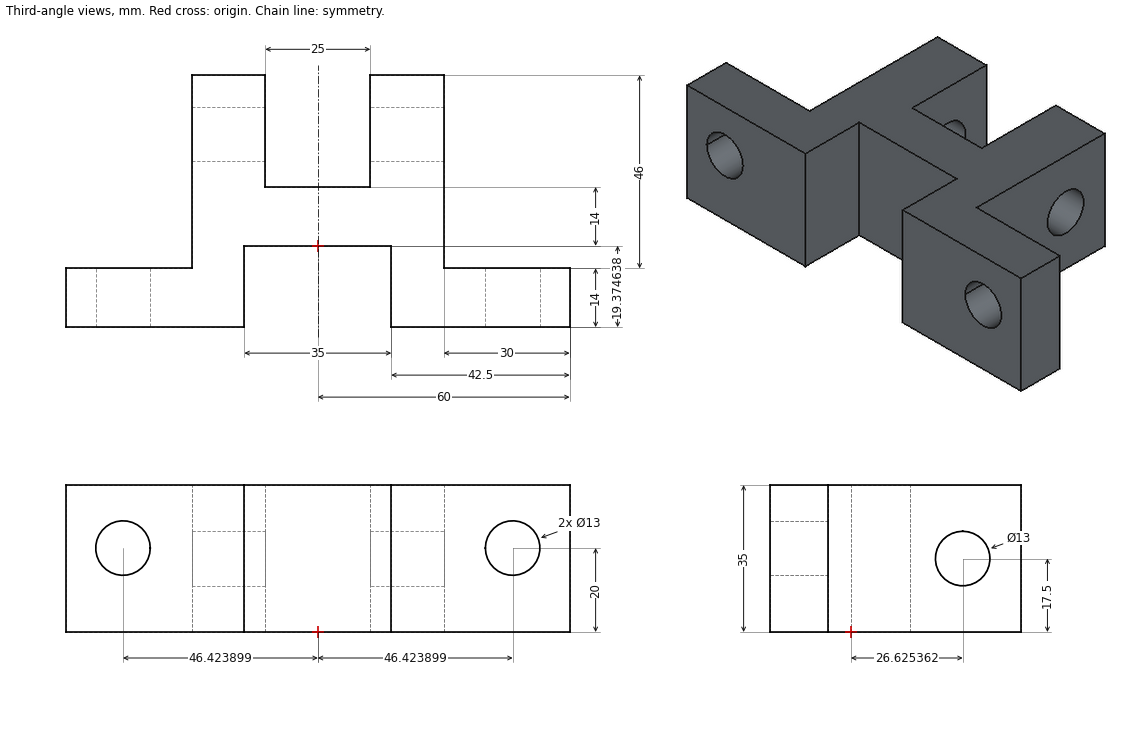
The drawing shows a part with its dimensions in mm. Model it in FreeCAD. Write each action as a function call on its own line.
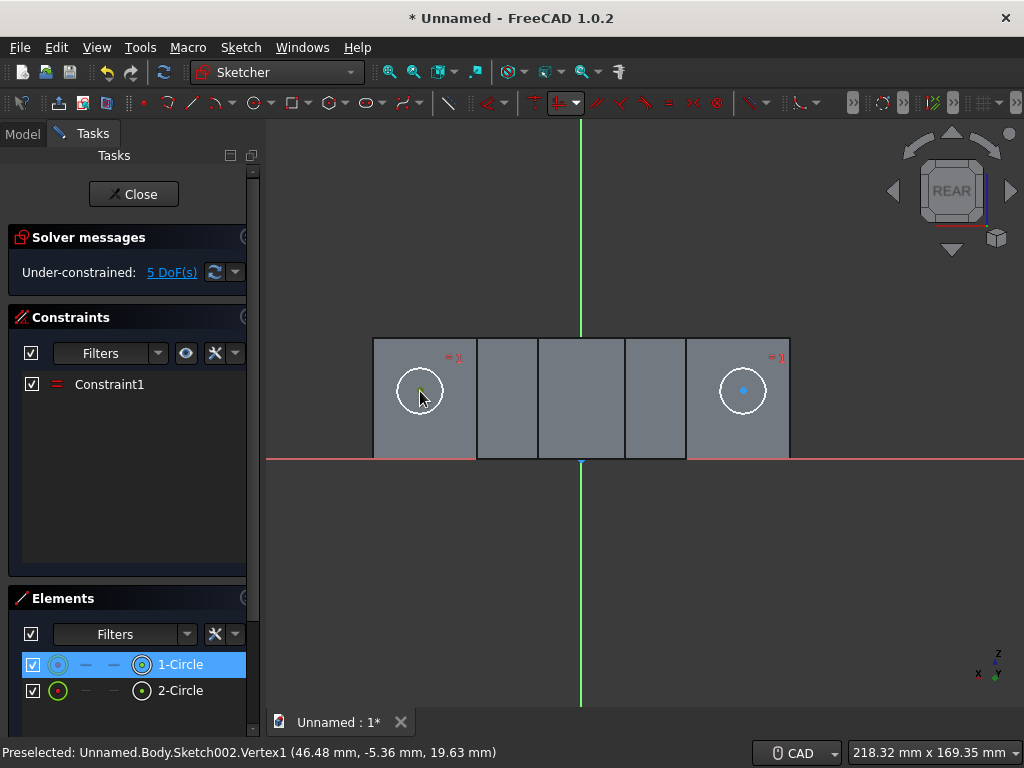
click(743, 391)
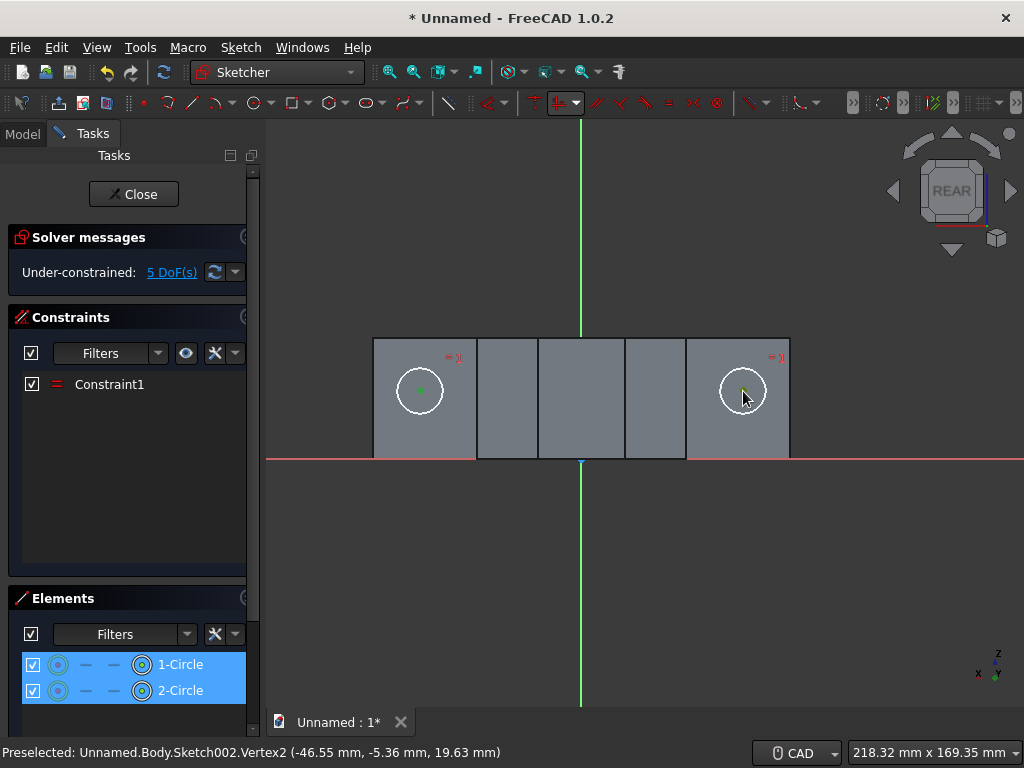
click(578, 104)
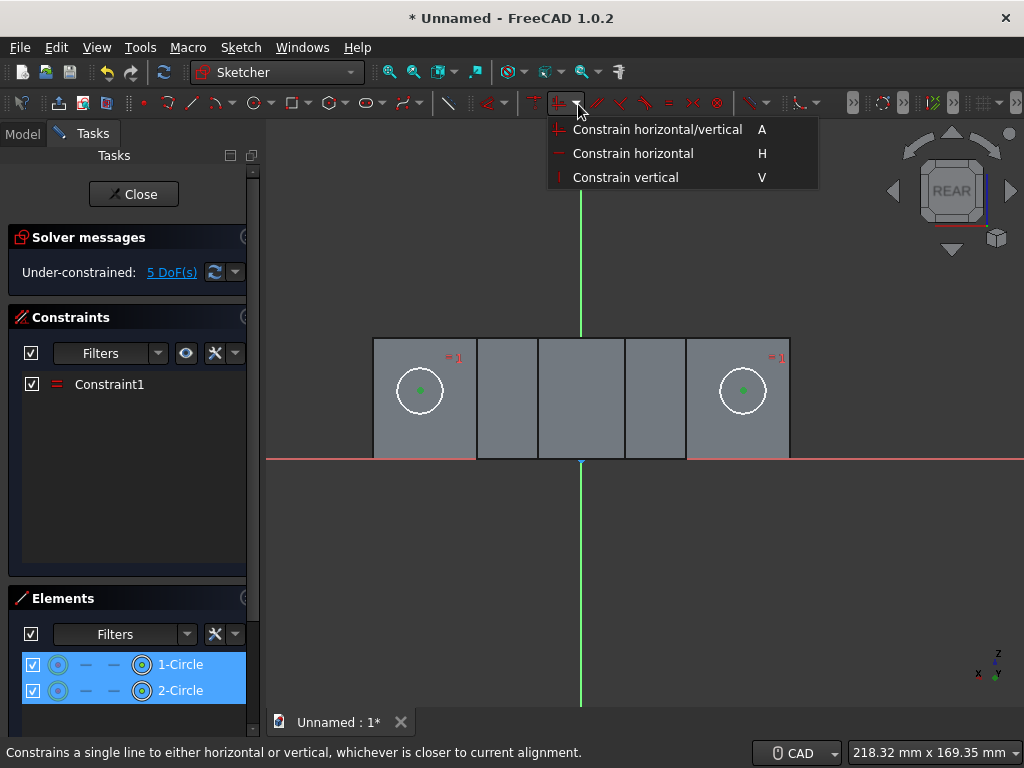
click(683, 153)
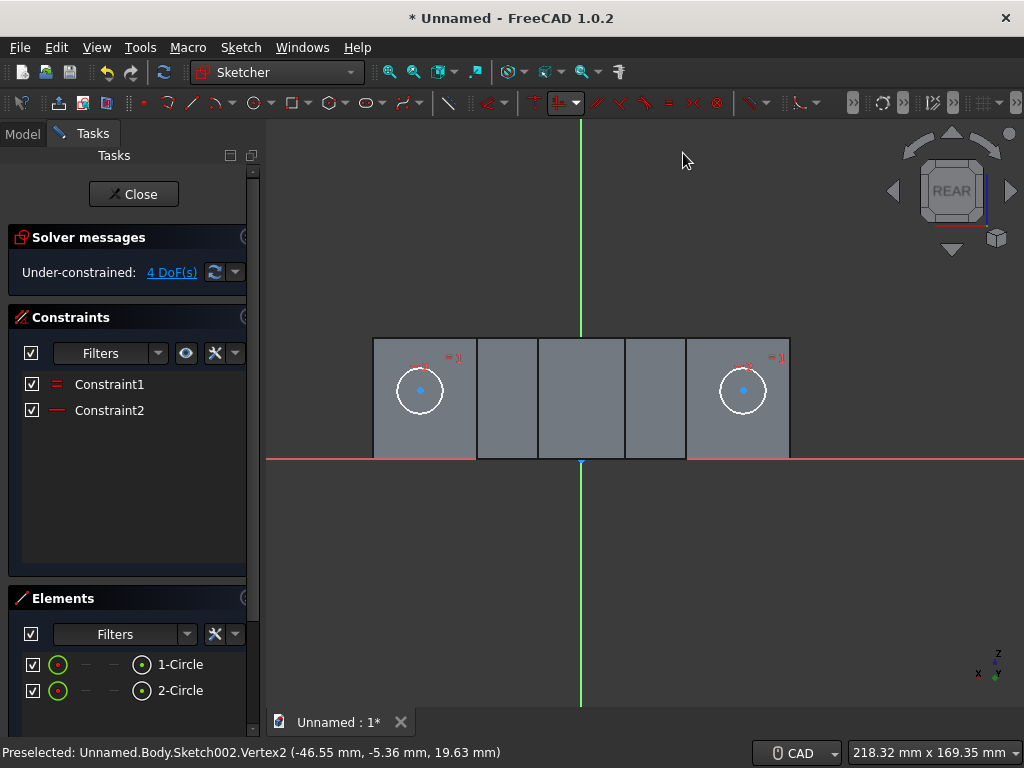
click(488, 104)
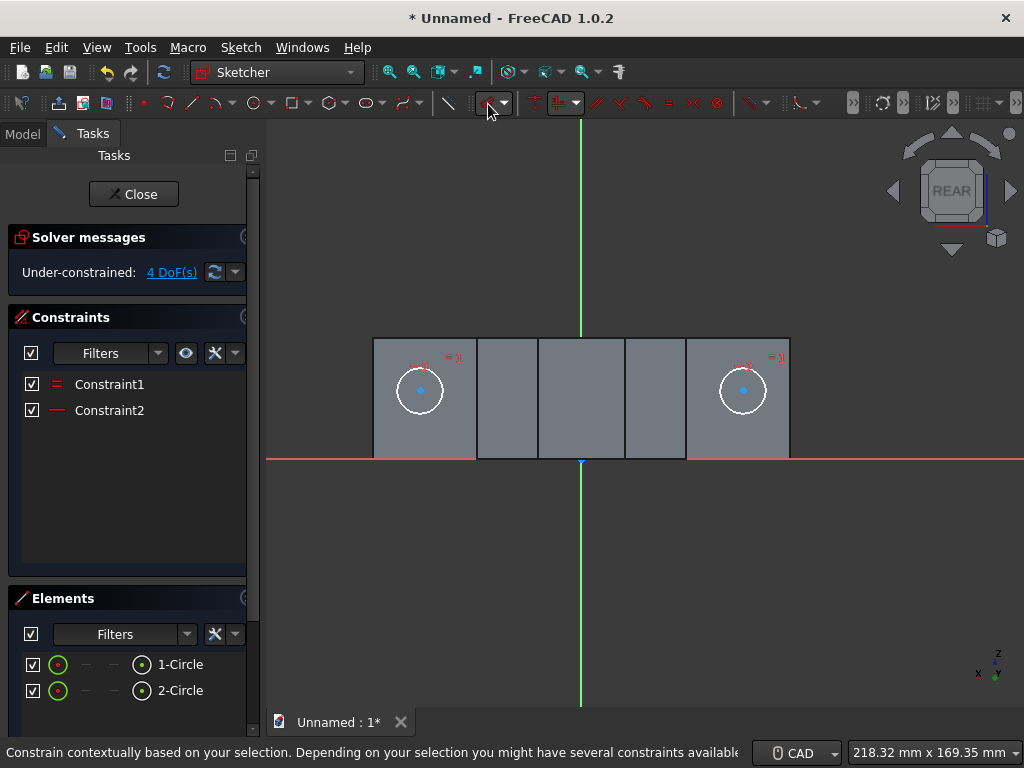
click(436, 375)
click(459, 352)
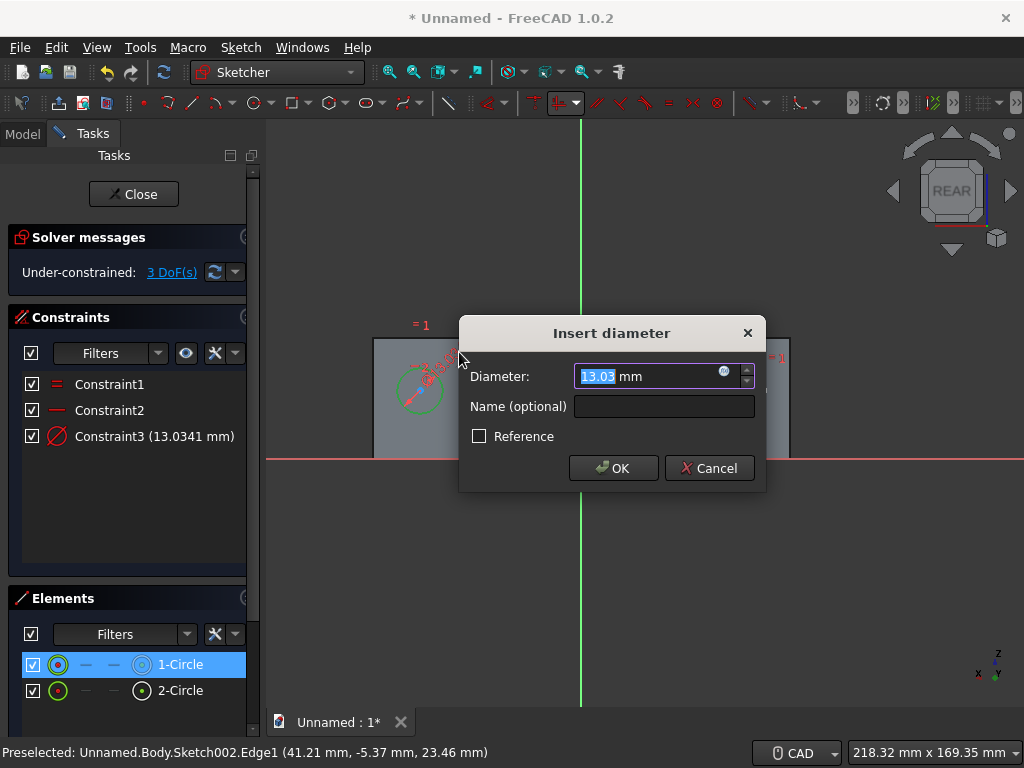
text(13)
key(Return)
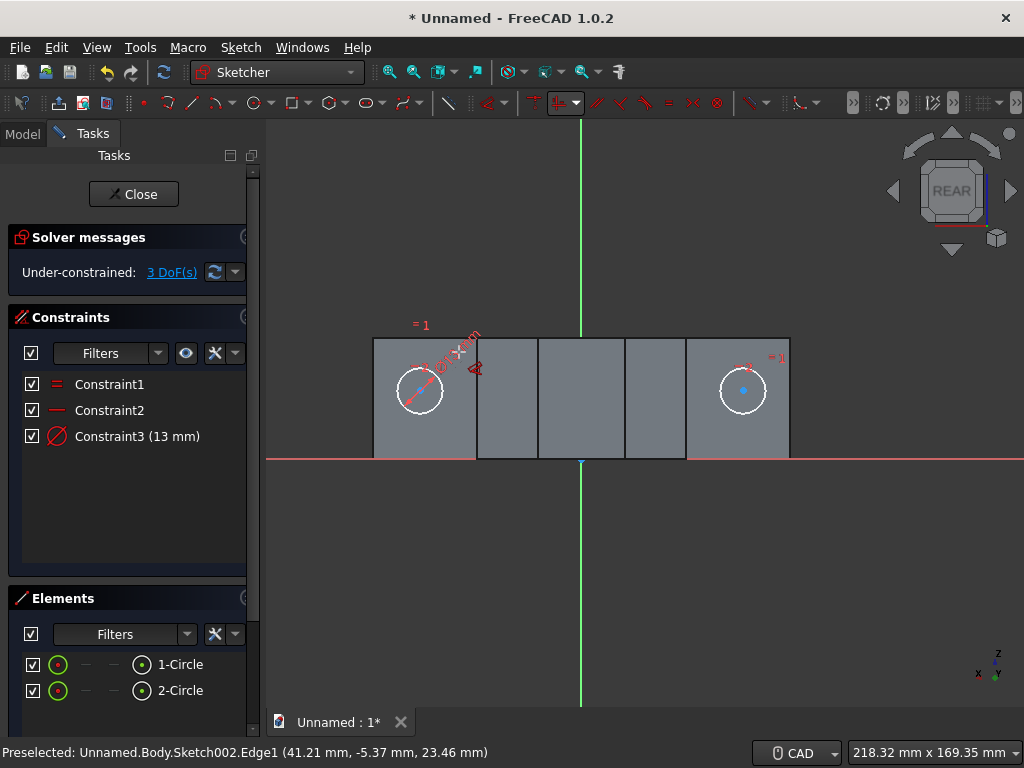
click(420, 391)
click(386, 425)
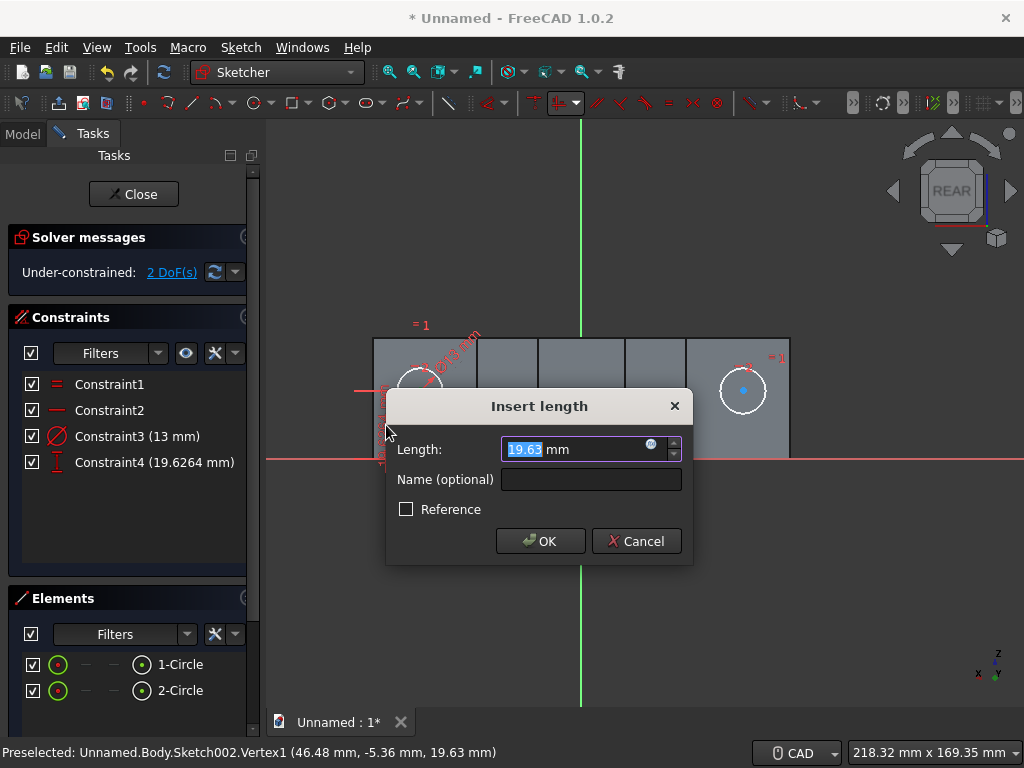
text(20)
key(Return)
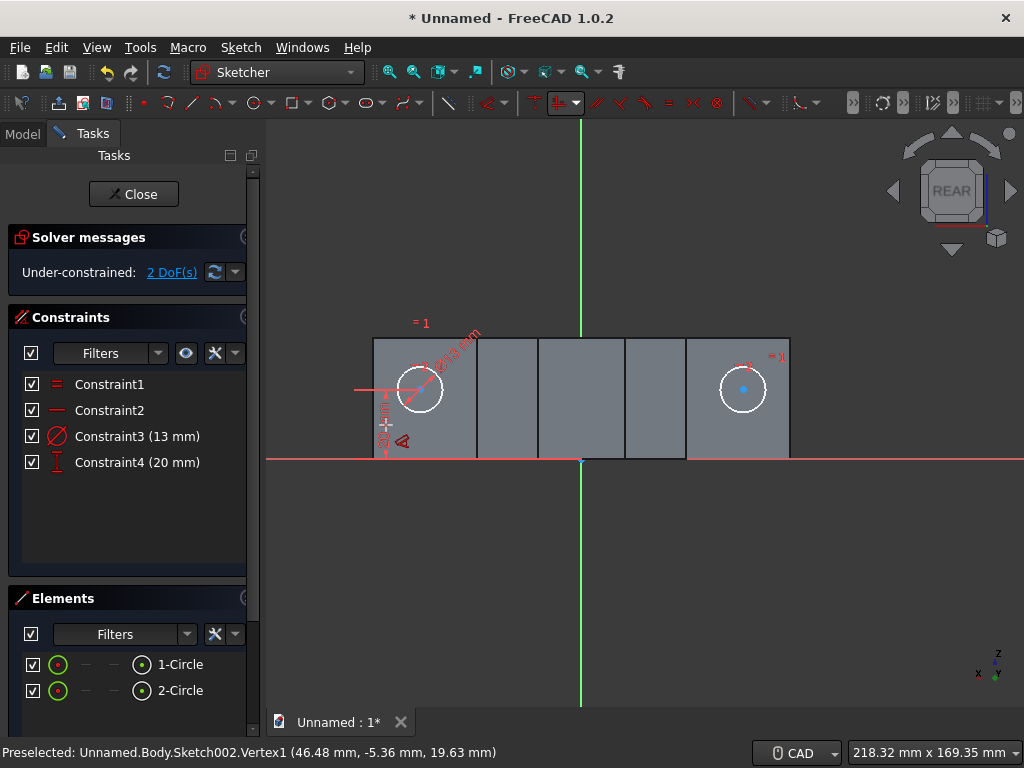
click(420, 390)
click(501, 493)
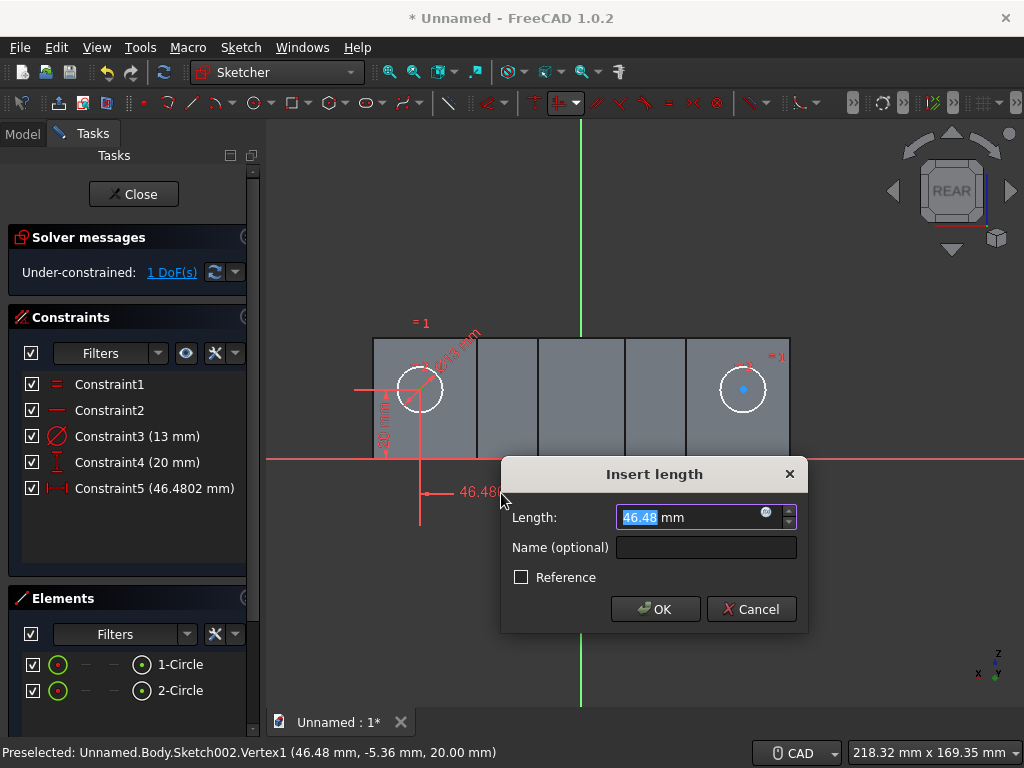
text(46.423899)
key(Return)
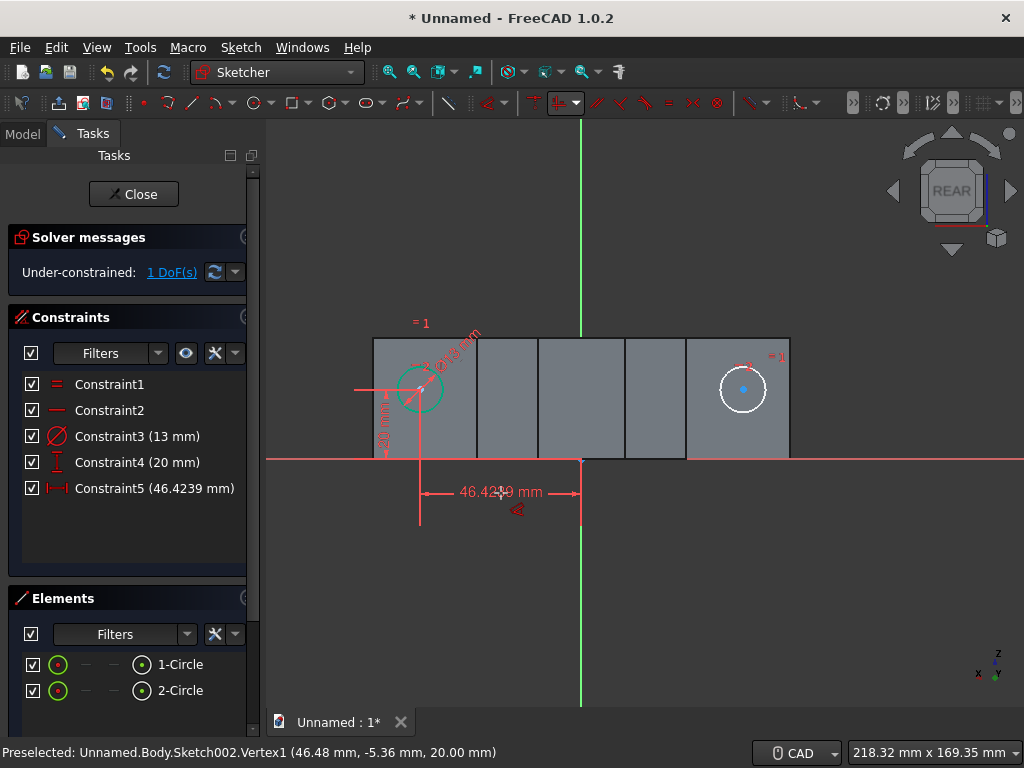
click(743, 390)
click(662, 493)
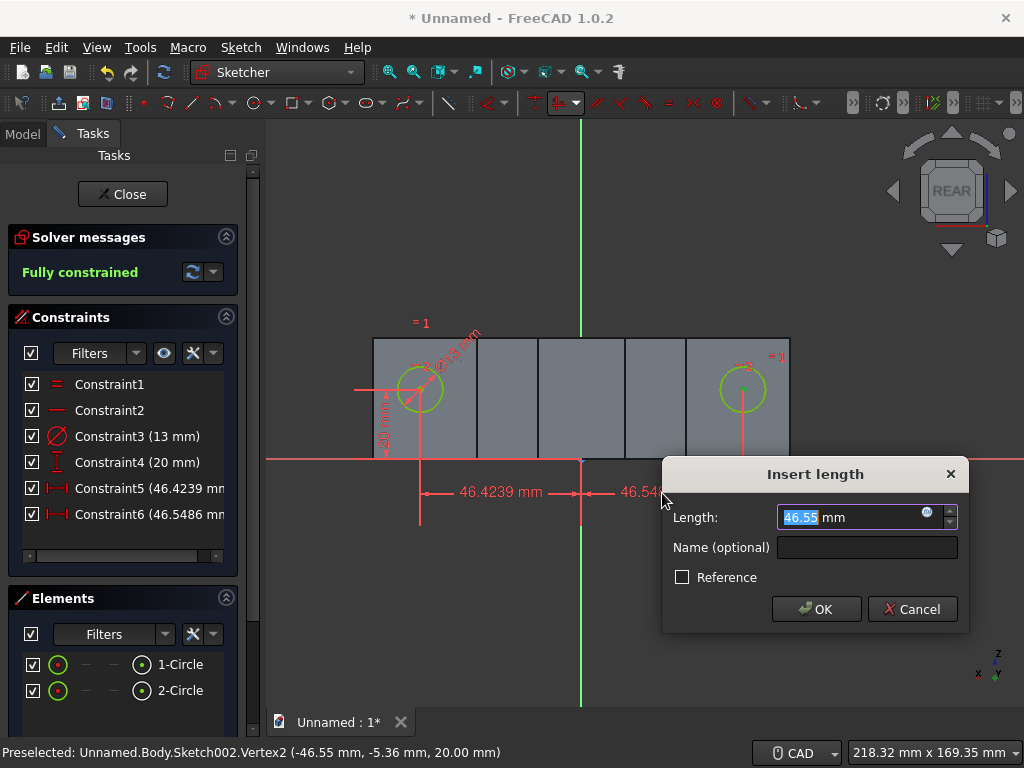
text(46.423899)
key(Return)
key(Escape)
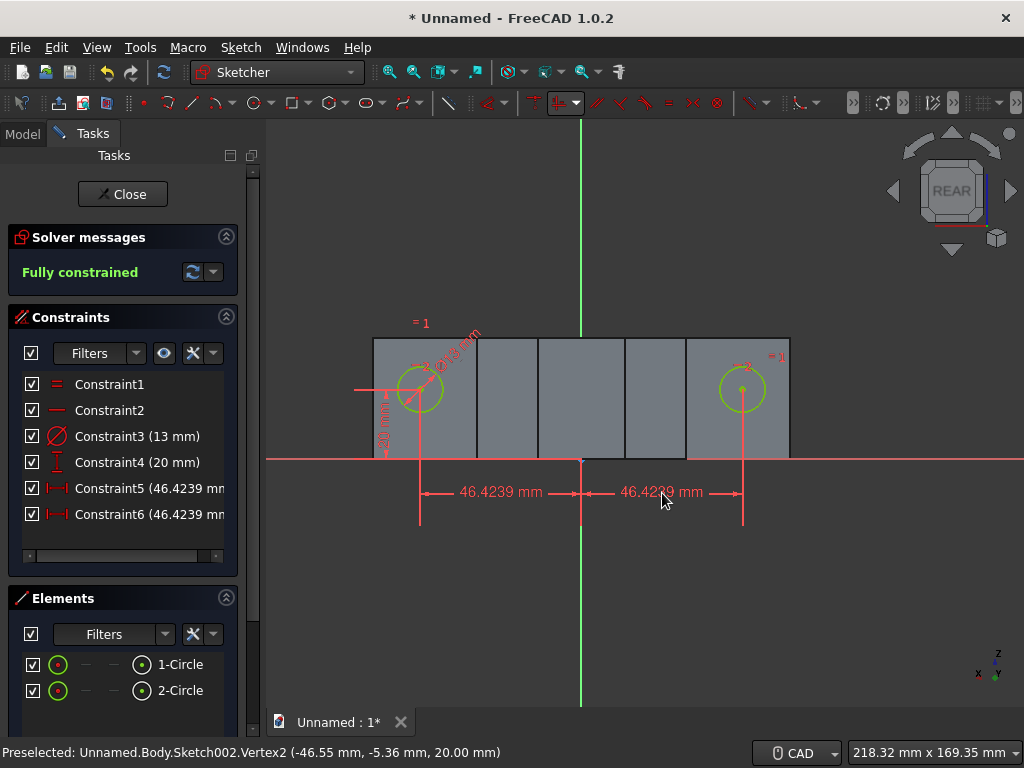
click(123, 194)